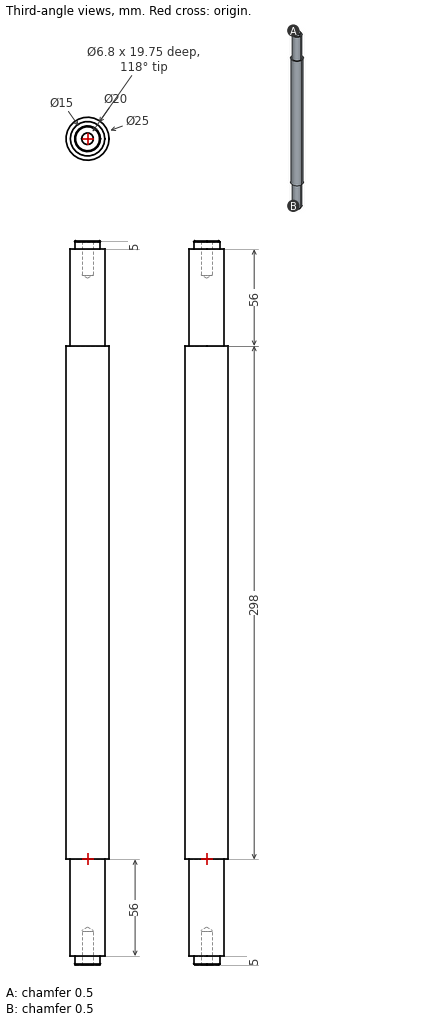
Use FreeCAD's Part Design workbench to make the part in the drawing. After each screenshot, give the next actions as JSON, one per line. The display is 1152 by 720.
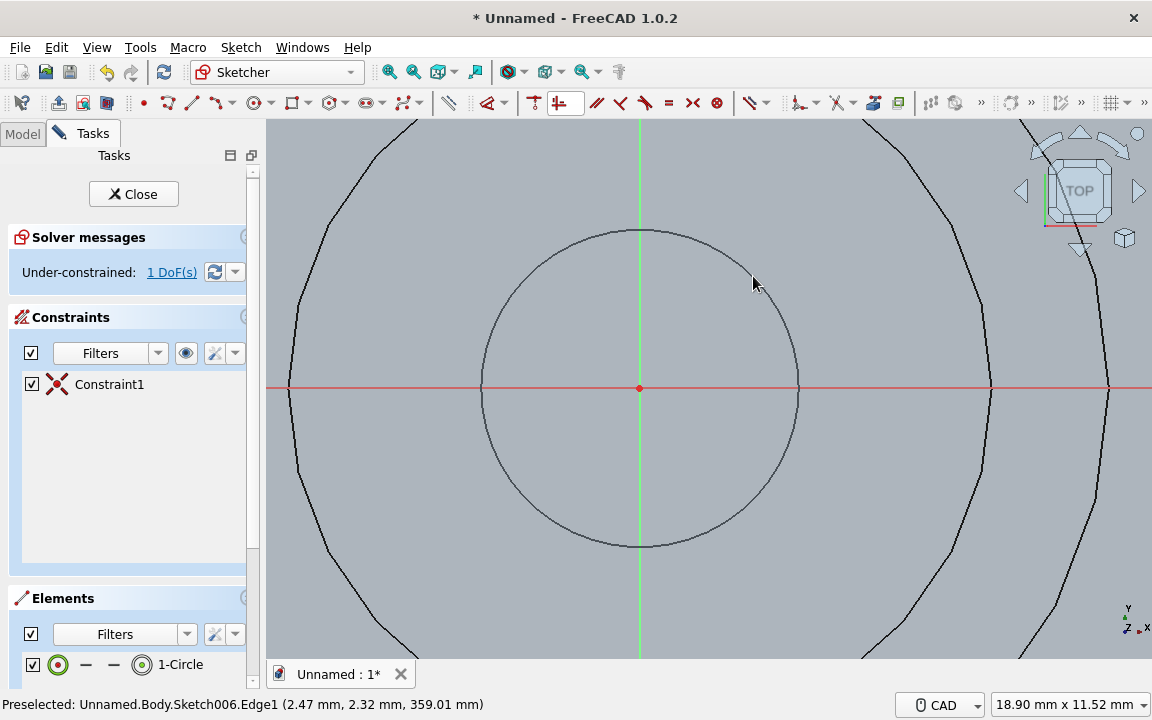
{"action": "left_click", "coordinate": [488, 104]}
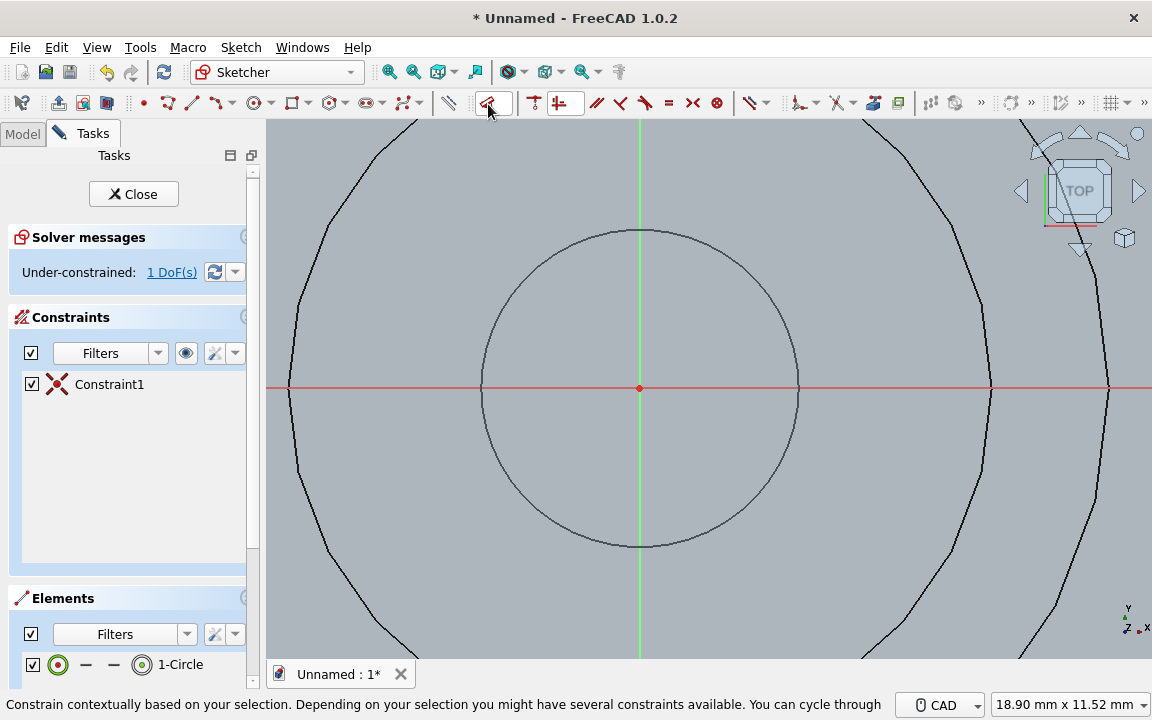
{"action": "left_click", "coordinate": [752, 276]}
{"action": "left_click", "coordinate": [775, 253]}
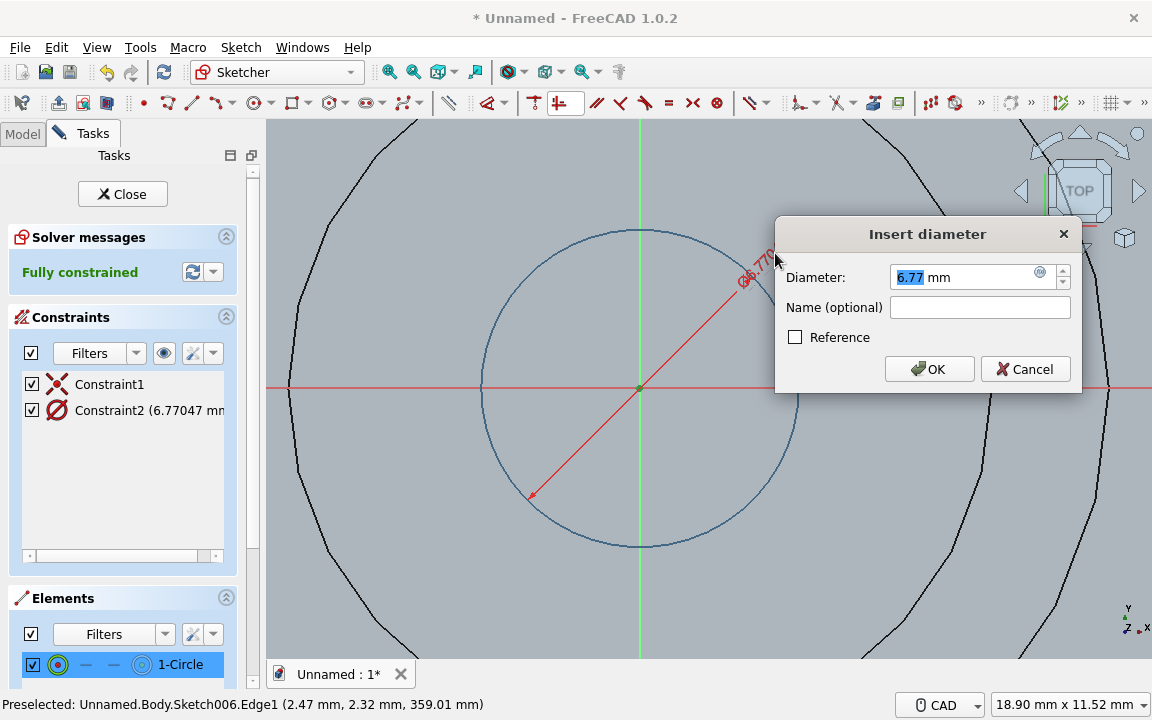
{"action": "type", "text": "6.8"}
{"action": "key", "text": "Return"}
{"action": "key", "text": "Escape"}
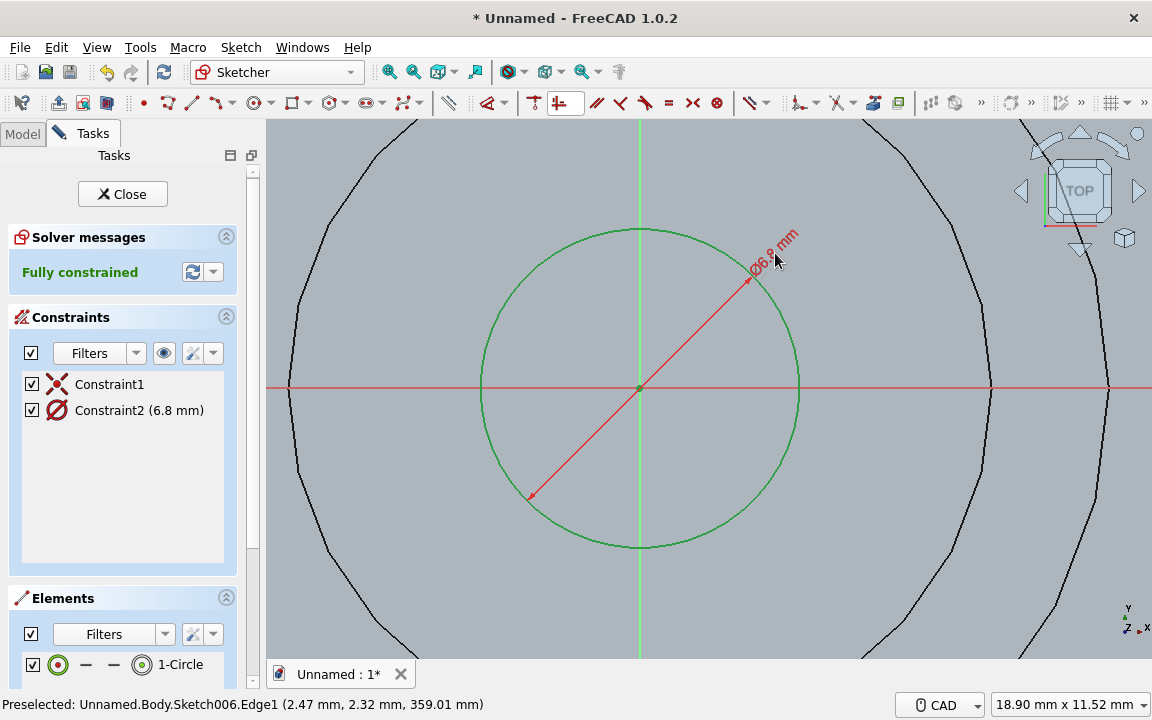
{"action": "left_click", "coordinate": [123, 194]}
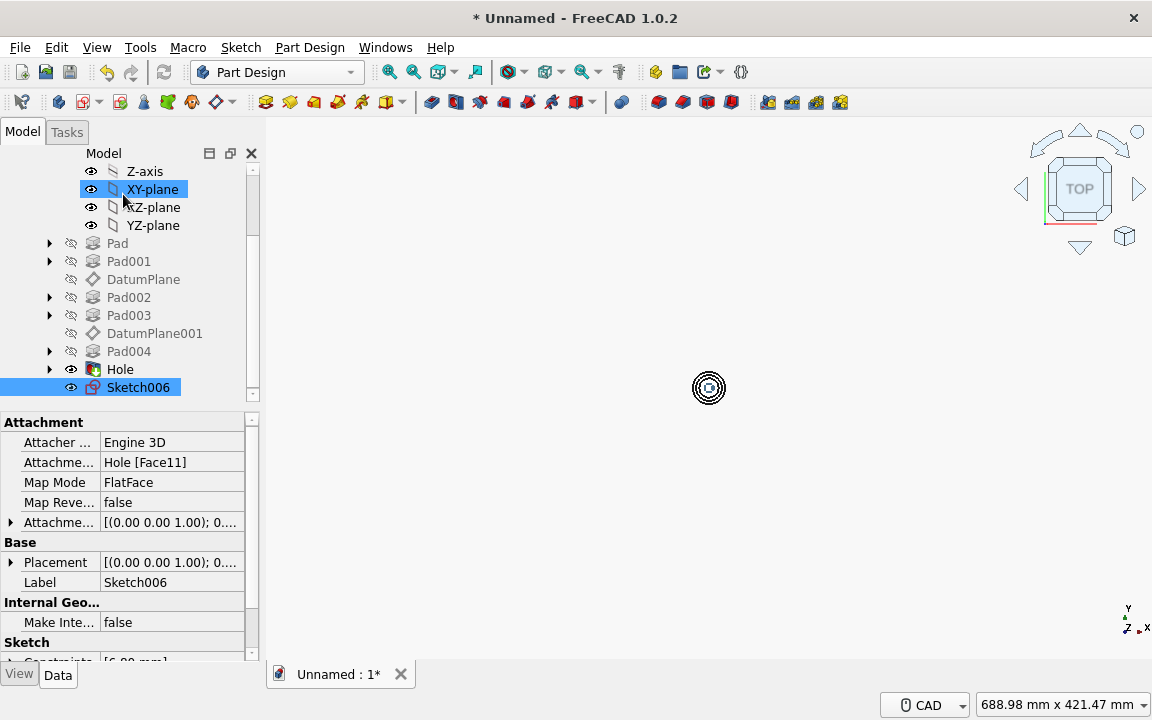
{"action": "left_click", "coordinate": [456, 102]}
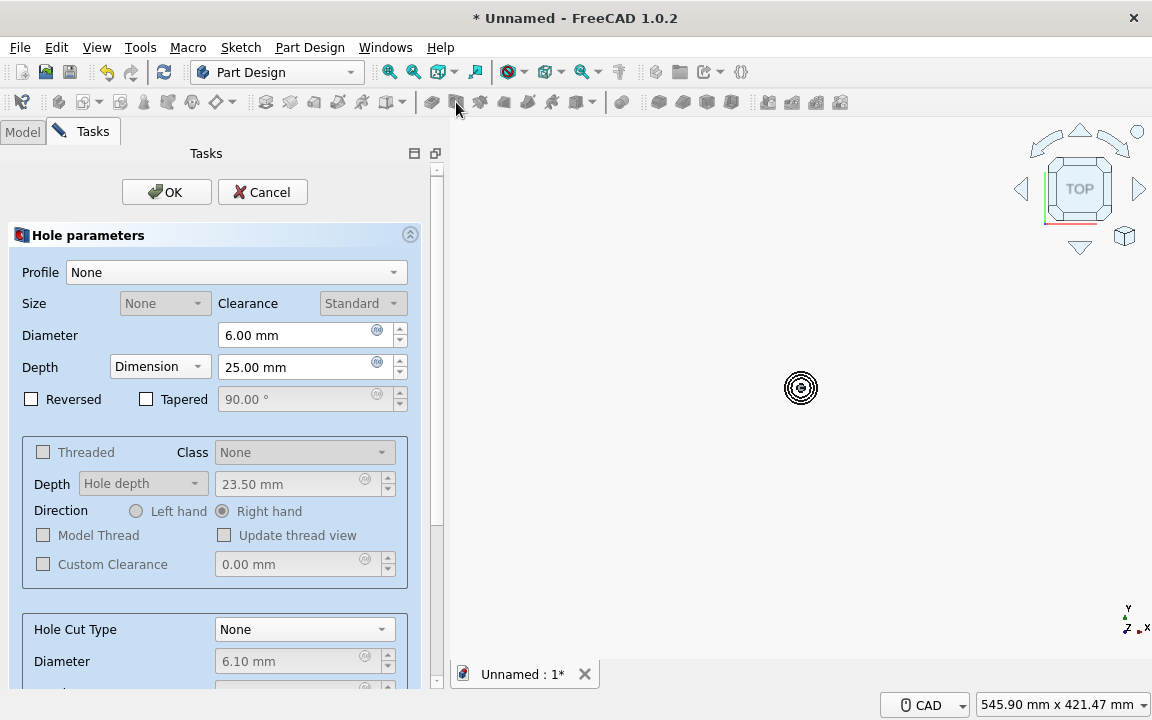
{"action": "triple_click", "coordinate": [305, 335]}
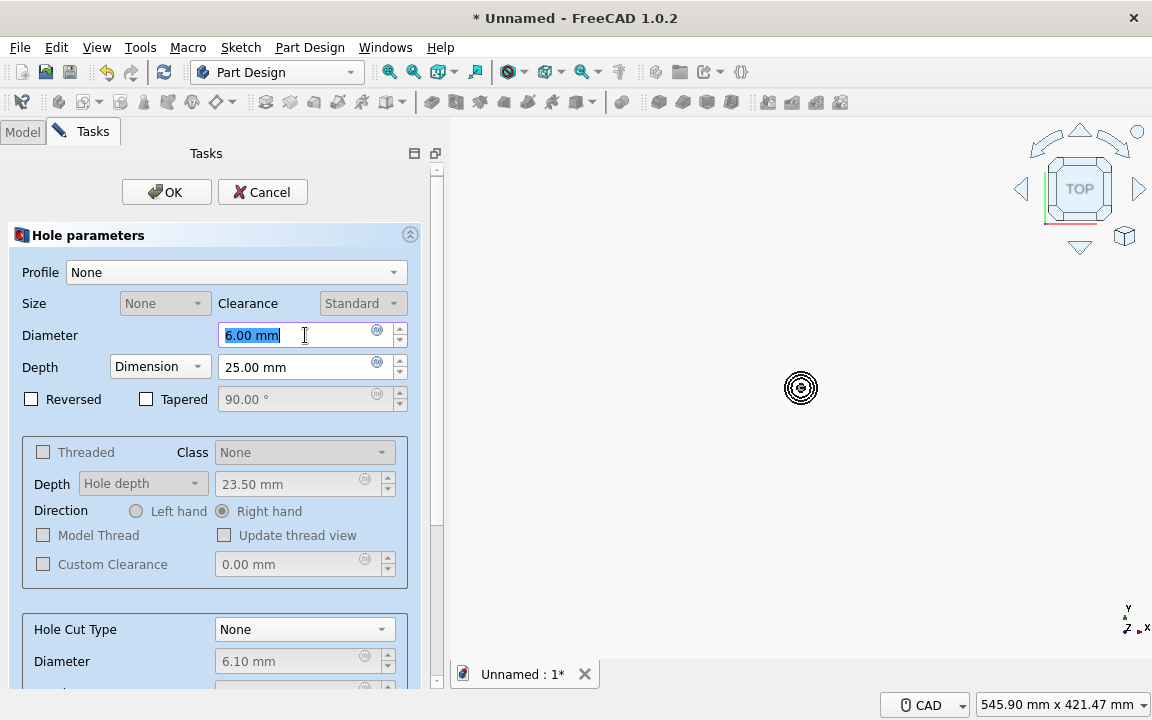
{"action": "type", "text": "6.8"}
{"action": "key", "text": "Tab"}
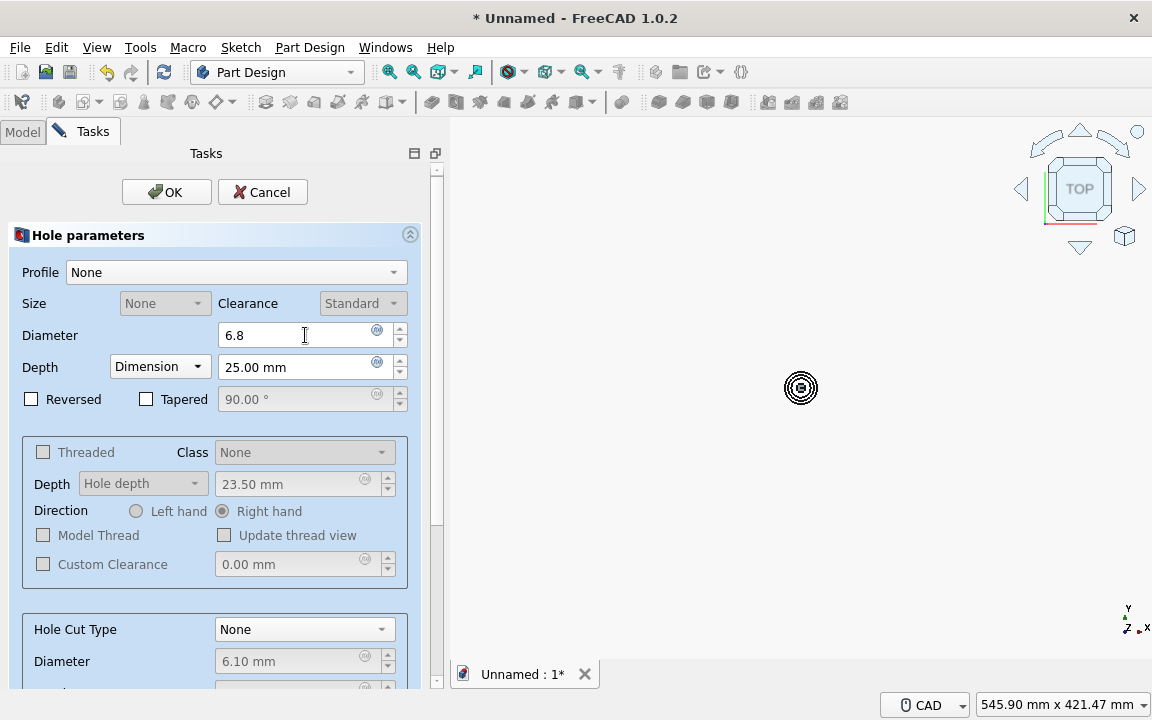
{"action": "triple_click", "coordinate": [305, 367]}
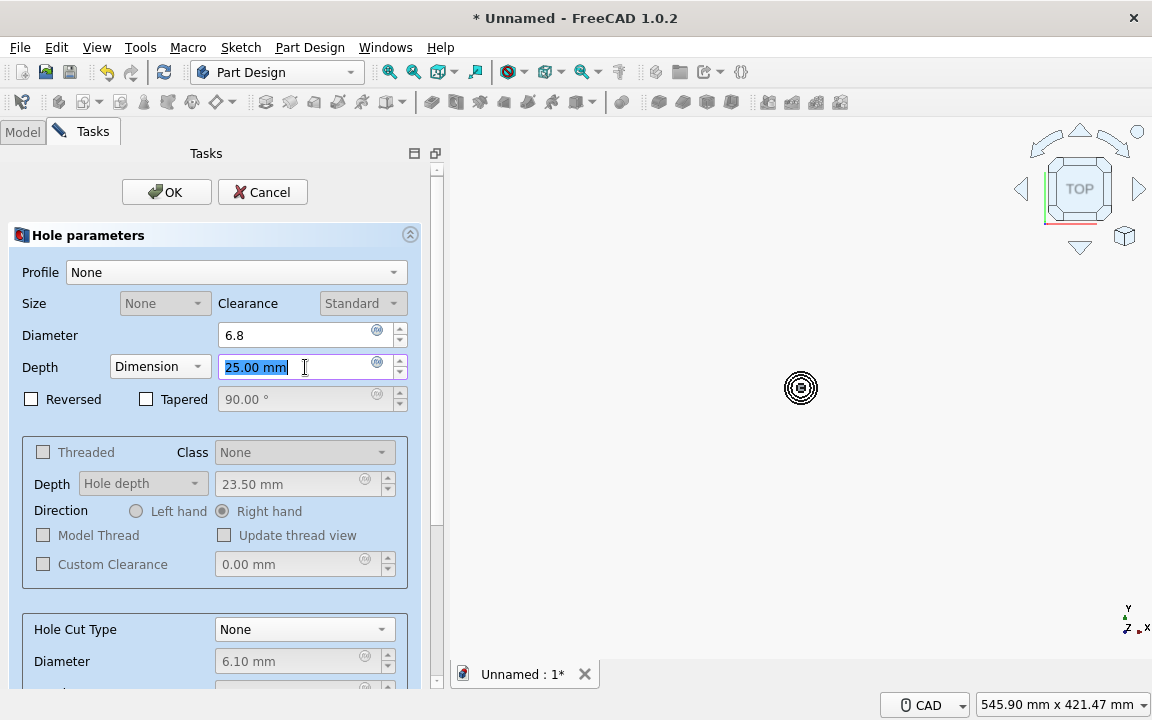
{"action": "type", "text": "19.75"}
{"action": "key", "text": "Tab"}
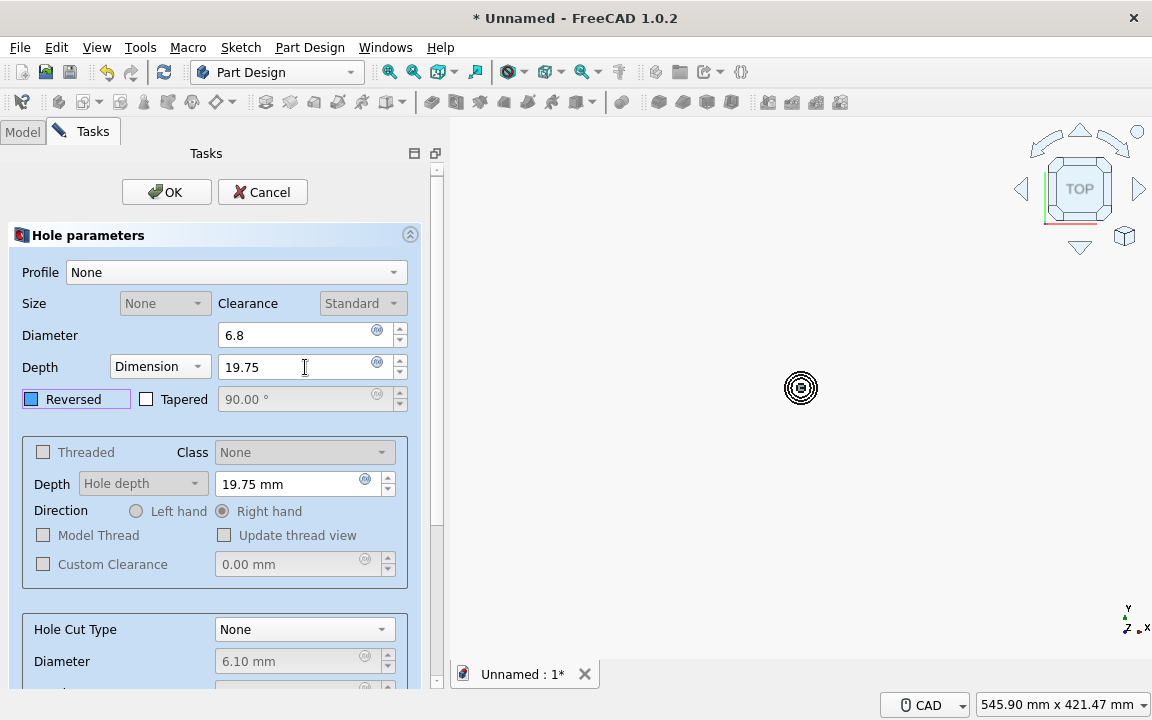
{"action": "left_click", "coordinate": [167, 192]}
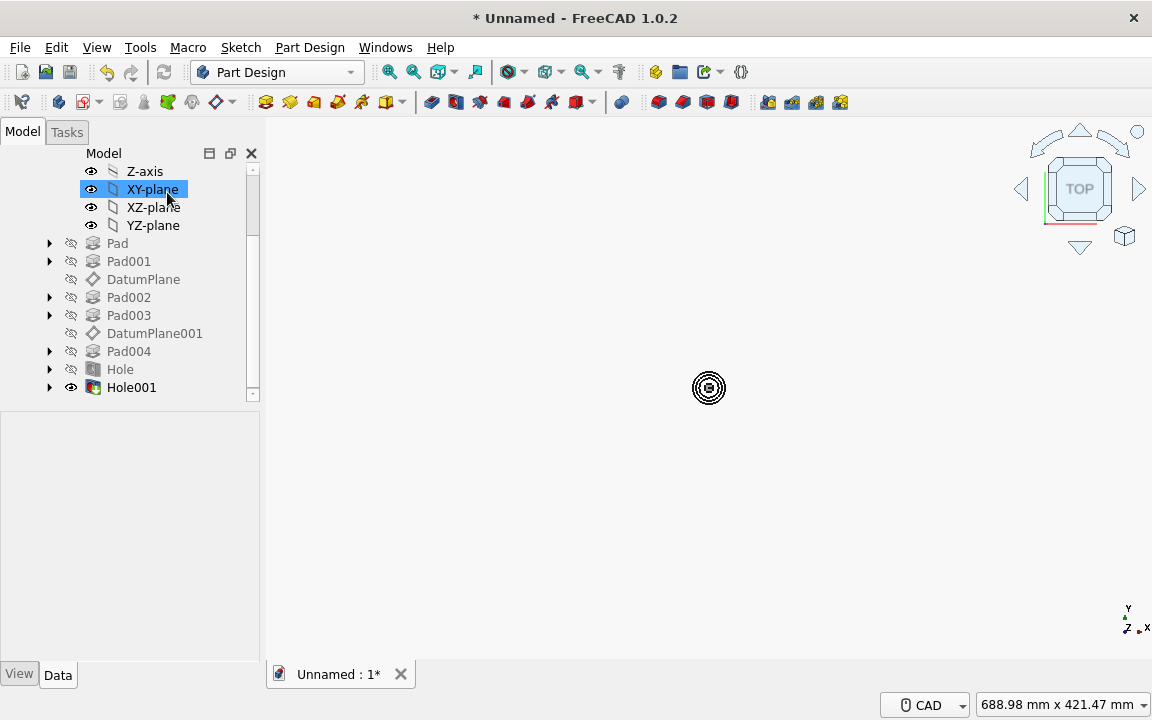
{"action": "left_click", "coordinate": [390, 72]}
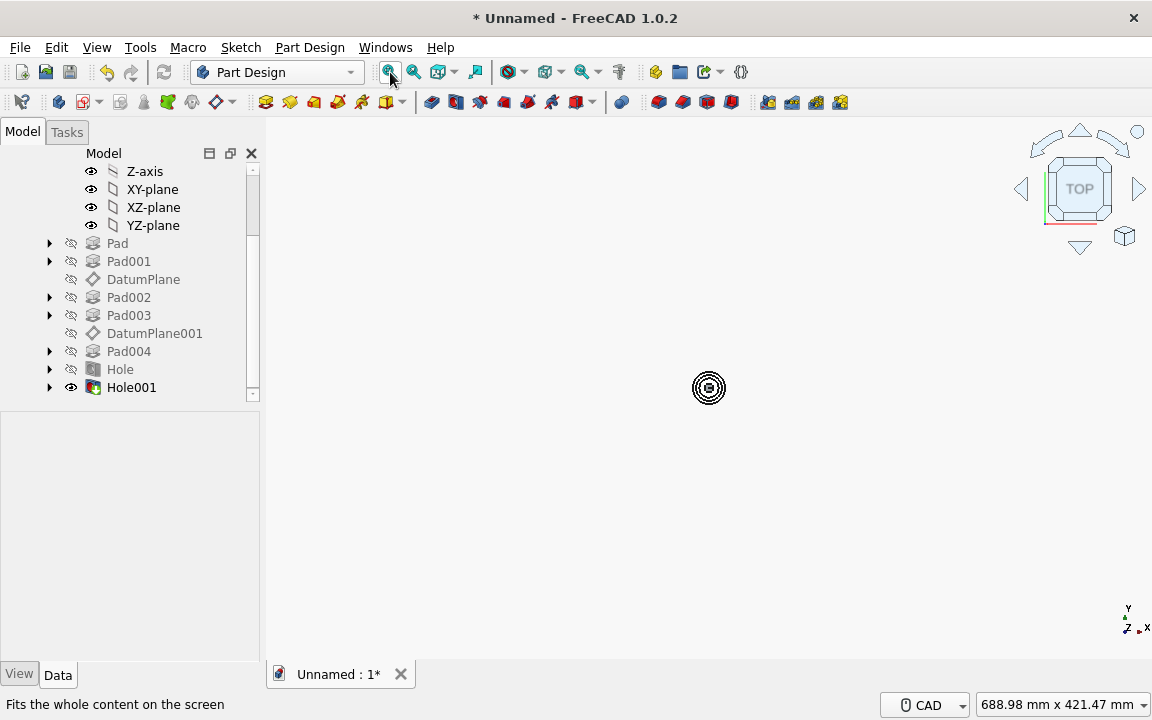
{"action": "left_click", "coordinate": [699, 387]}